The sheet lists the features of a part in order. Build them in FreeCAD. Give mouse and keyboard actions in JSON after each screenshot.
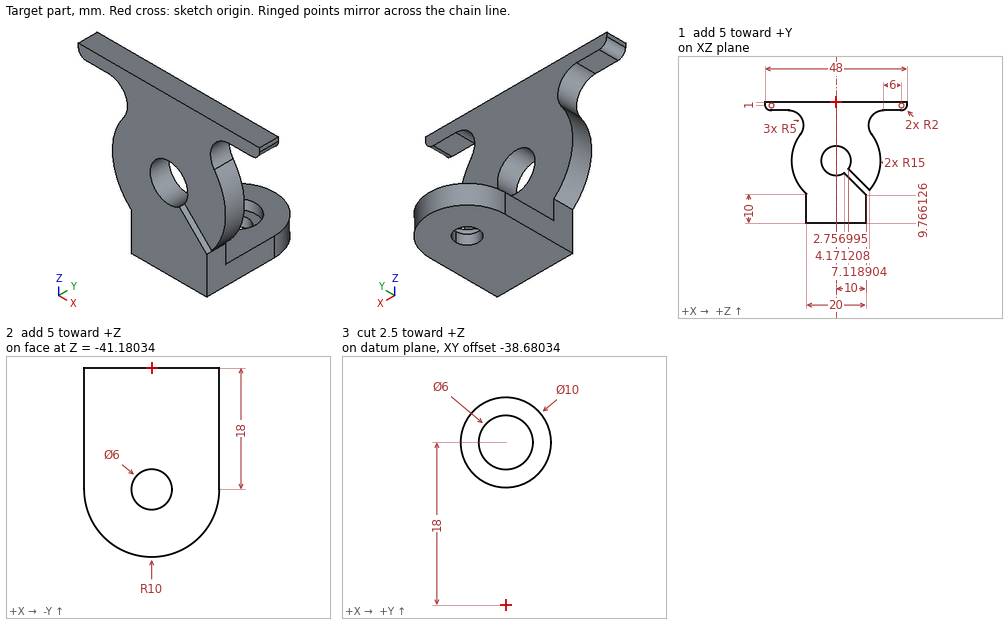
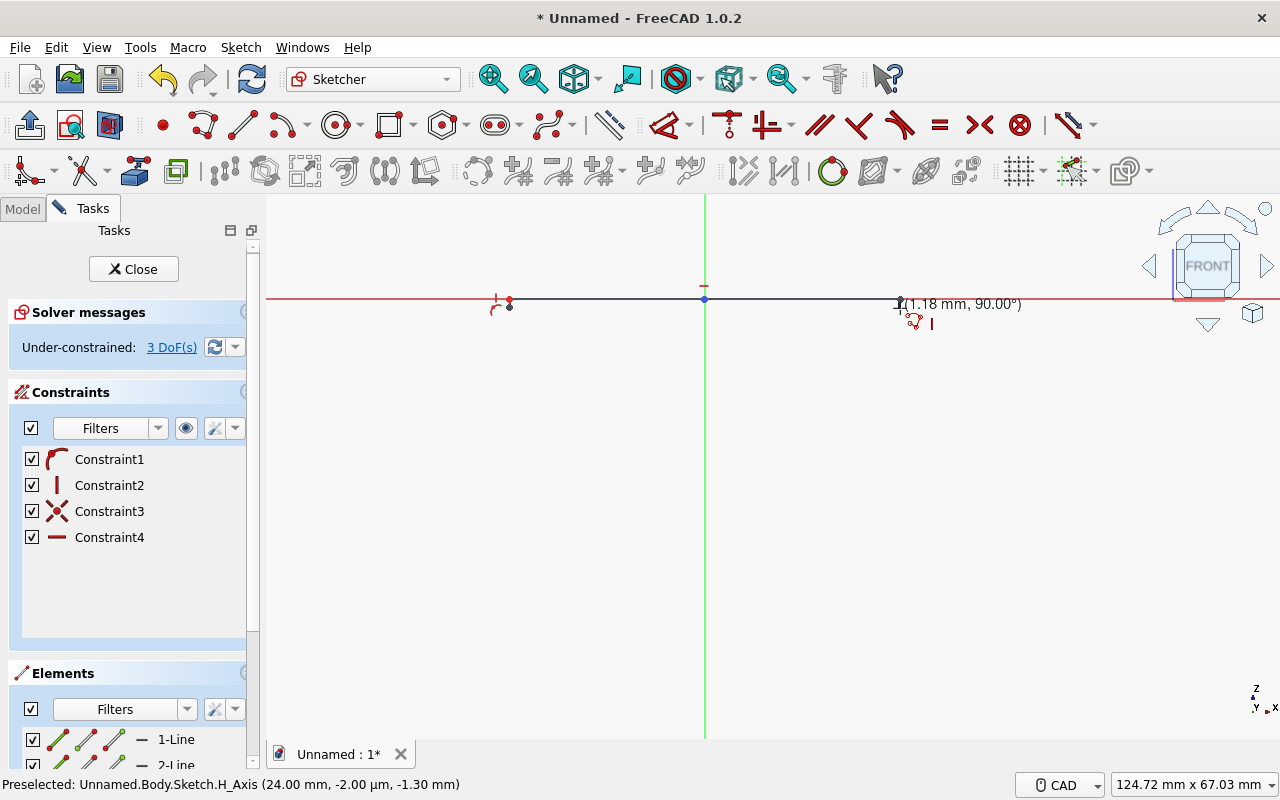
{"action": "scroll", "coordinate": [900, 308], "scroll_direction": "up", "scroll_amount": 4}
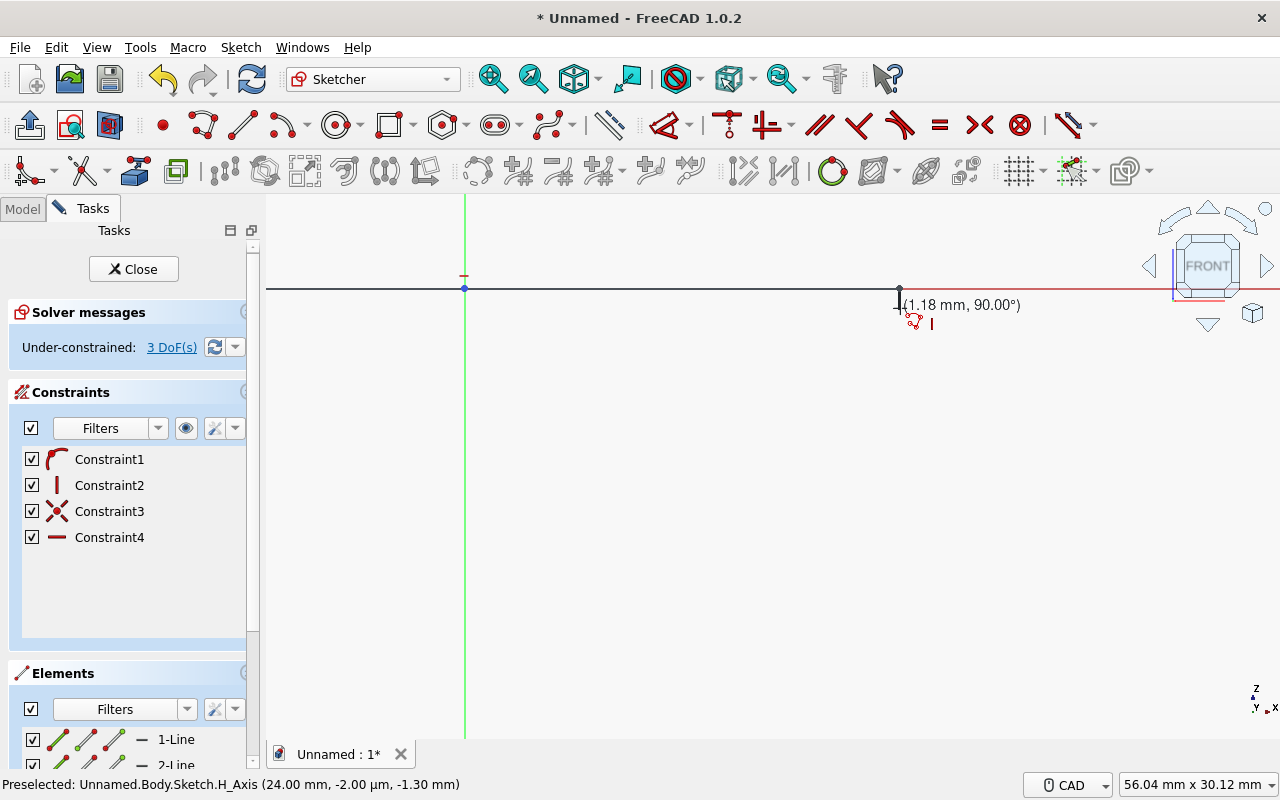
{"action": "left_click", "coordinate": [899, 307]}
{"action": "right_click", "coordinate": [899, 307]}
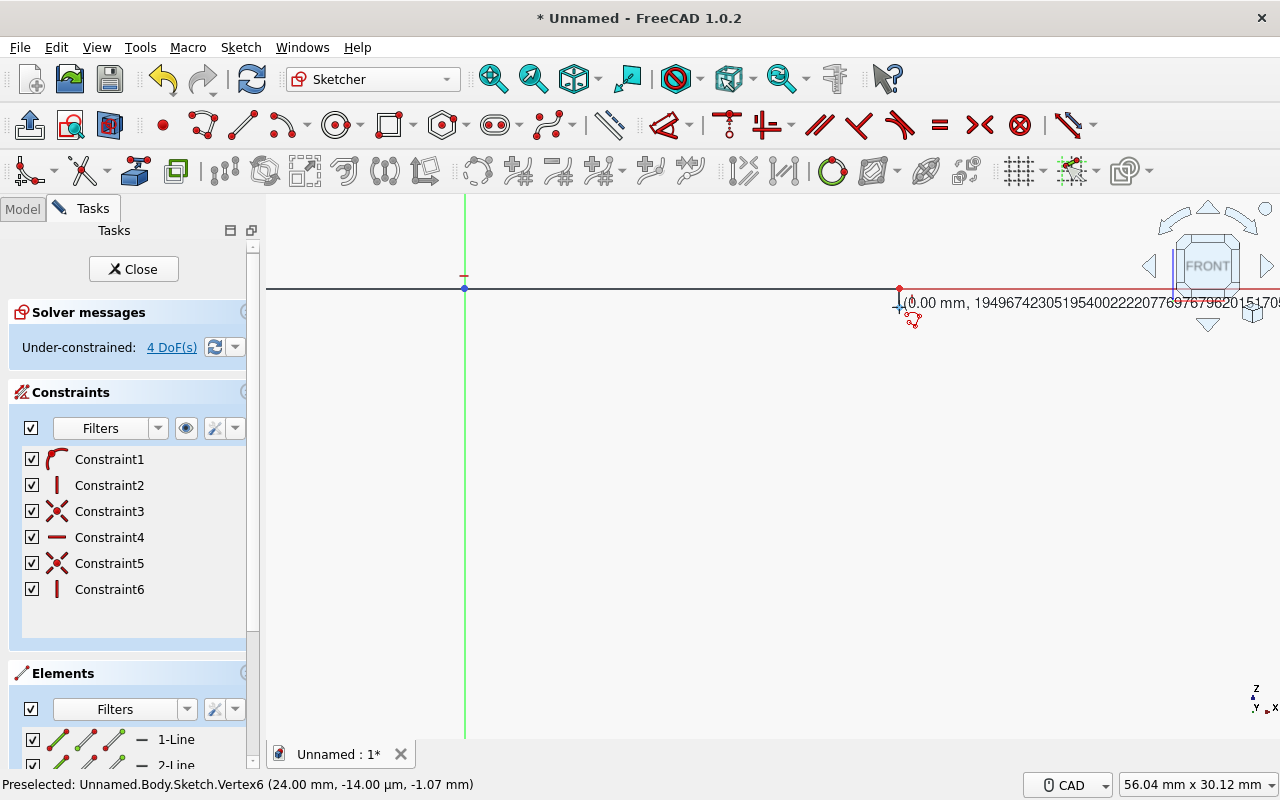
{"action": "key", "text": "g l"}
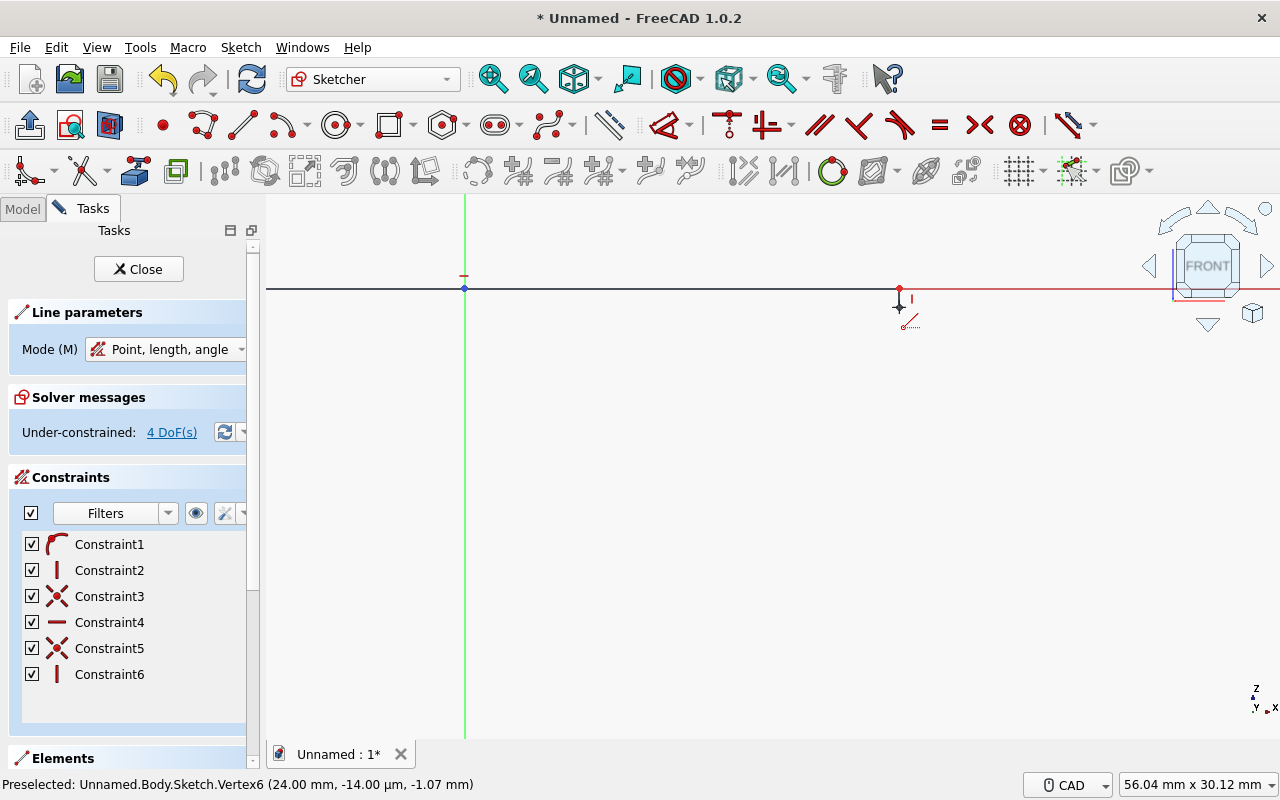
{"action": "left_click", "coordinate": [863, 343]}
{"action": "left_click", "coordinate": [754, 343]}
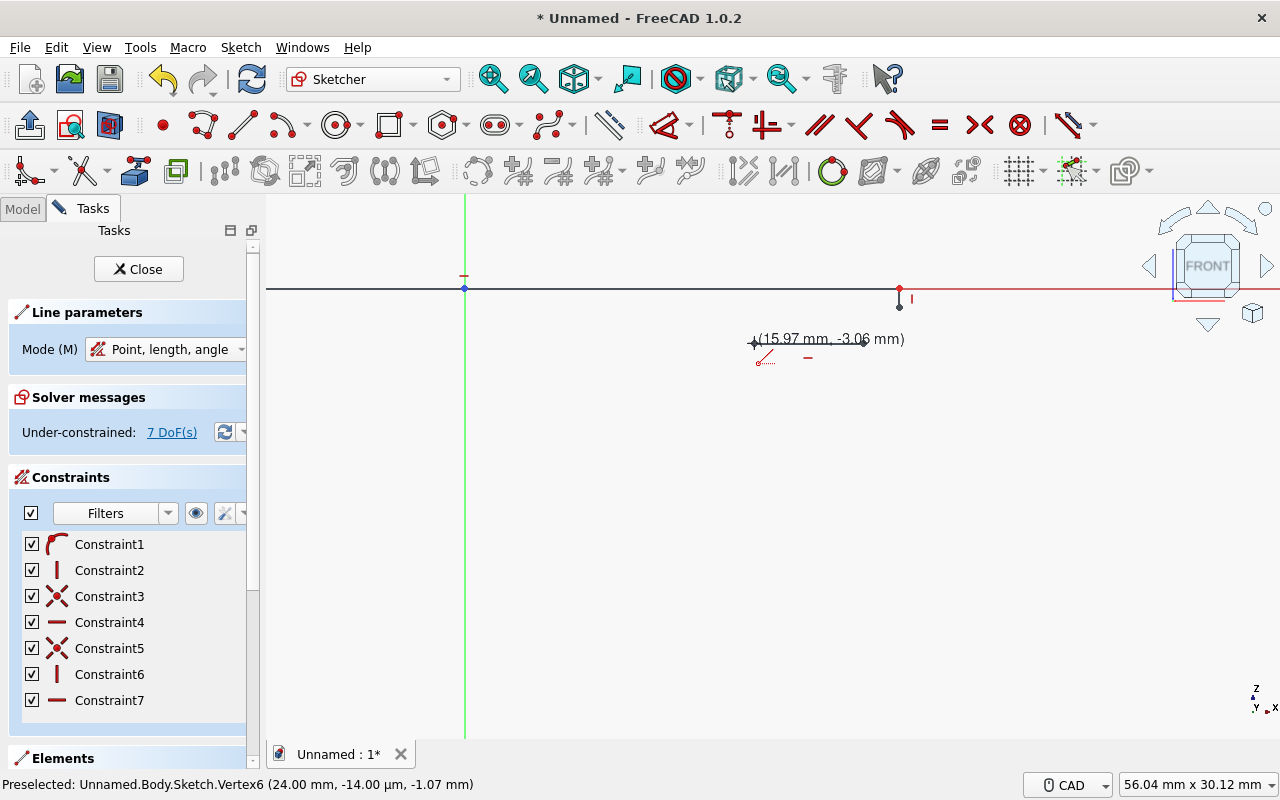
{"action": "scroll", "coordinate": [900, 308], "scroll_direction": "down", "scroll_amount": 4}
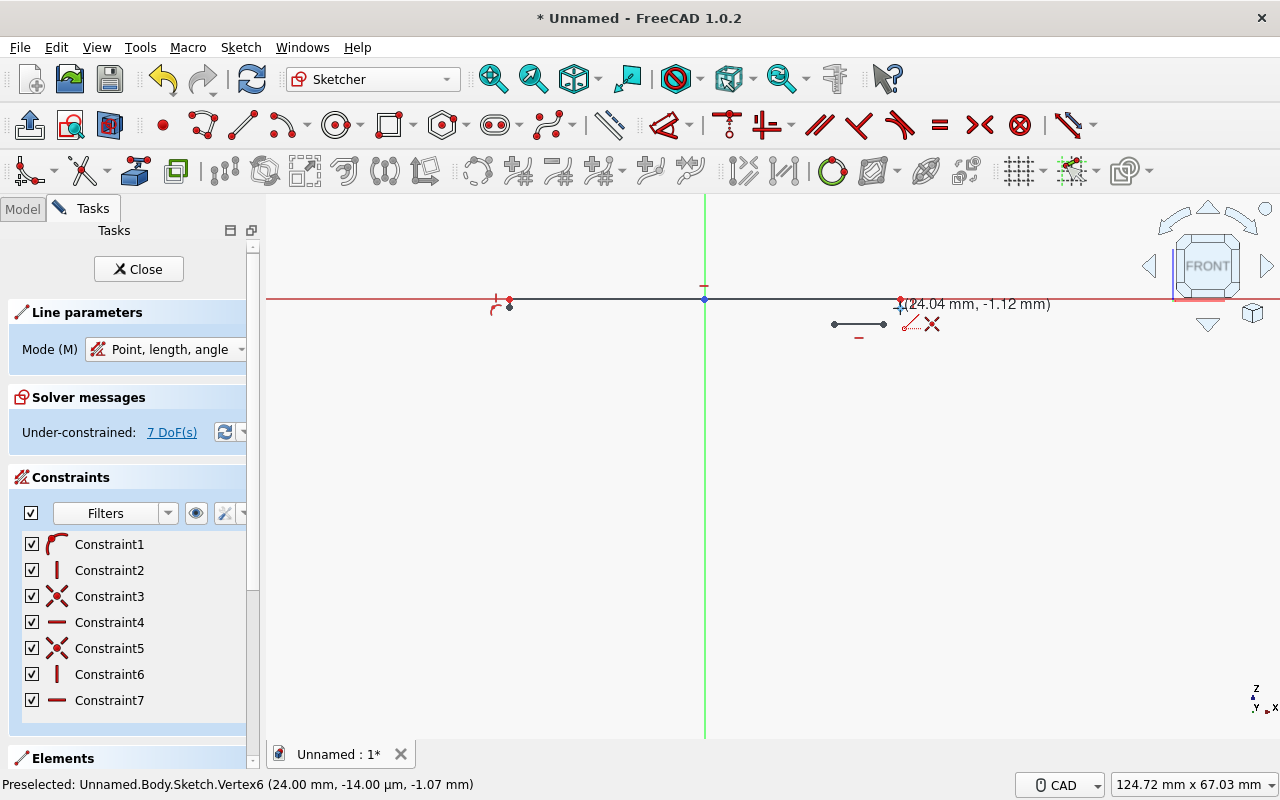
{"action": "left_click", "coordinate": [797, 542]}
{"action": "left_click", "coordinate": [739, 484]}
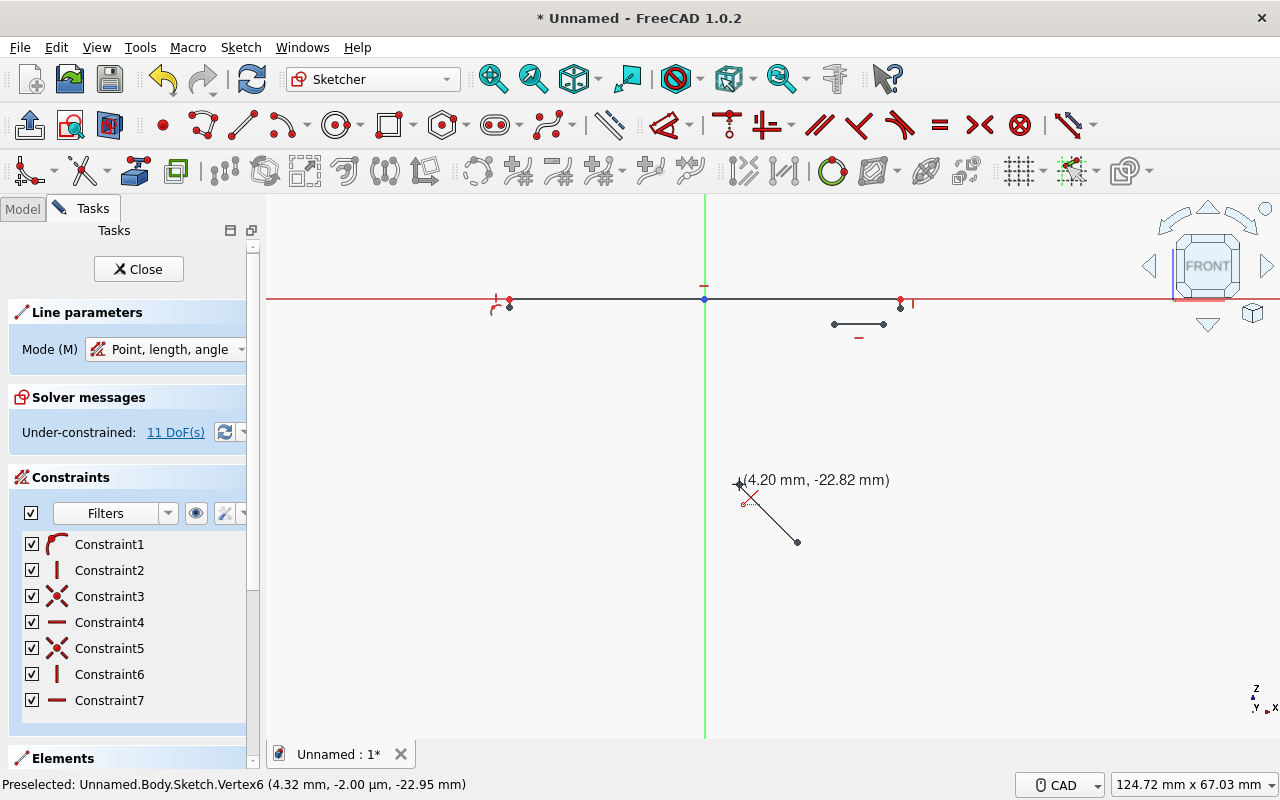
{"action": "key", "text": "g m"}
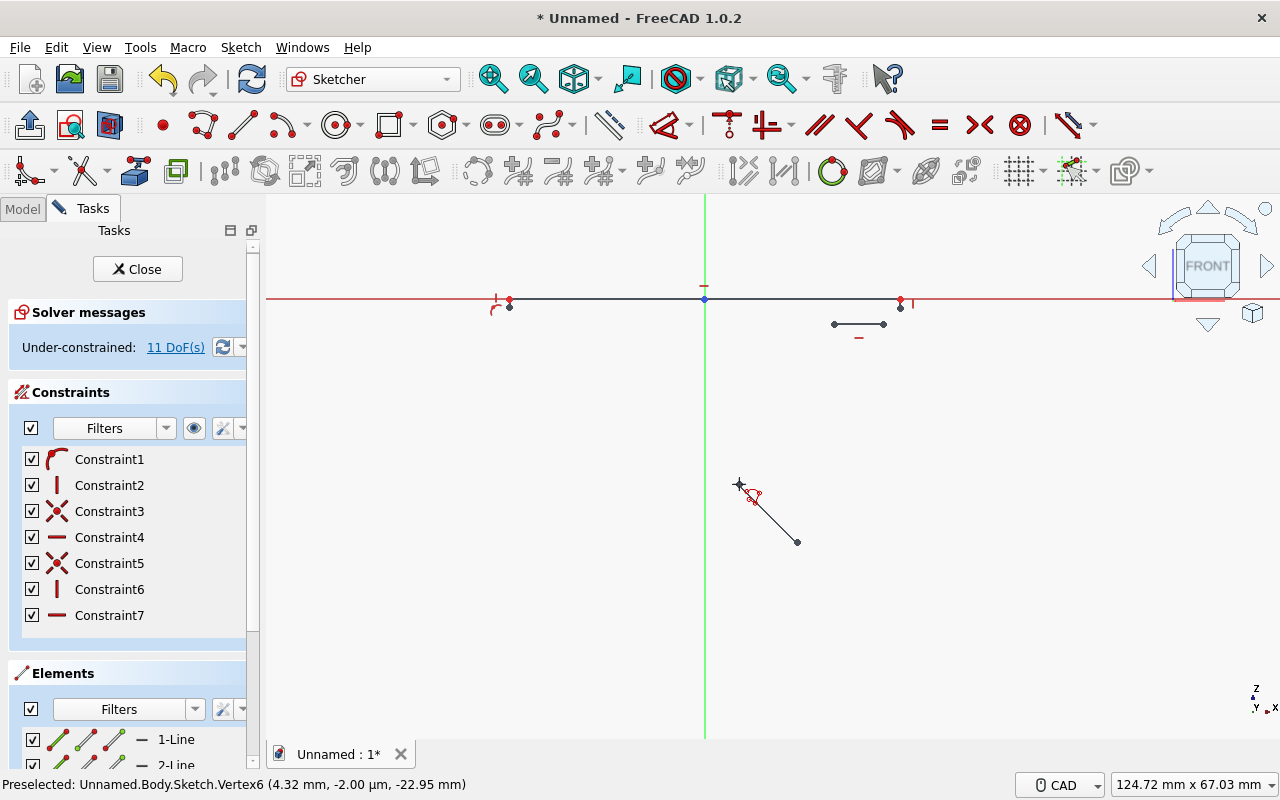
{"action": "left_click", "coordinate": [727, 496]}
{"action": "left_click", "coordinate": [786, 555]}
{"action": "left_click", "coordinate": [786, 634]}
{"action": "left_click", "coordinate": [624, 634]}
{"action": "left_click", "coordinate": [624, 553]}
{"action": "right_click", "coordinate": [624, 553]}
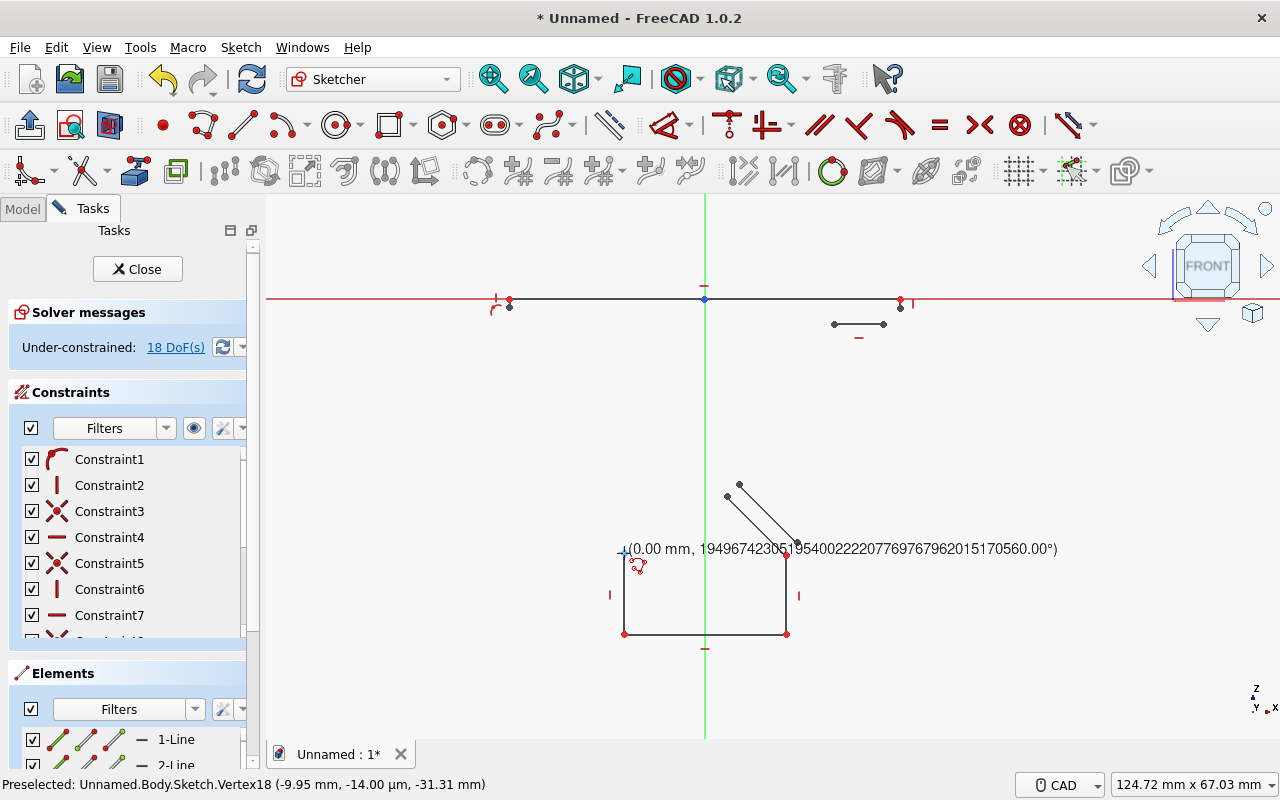
{"action": "left_click", "coordinate": [244, 126]}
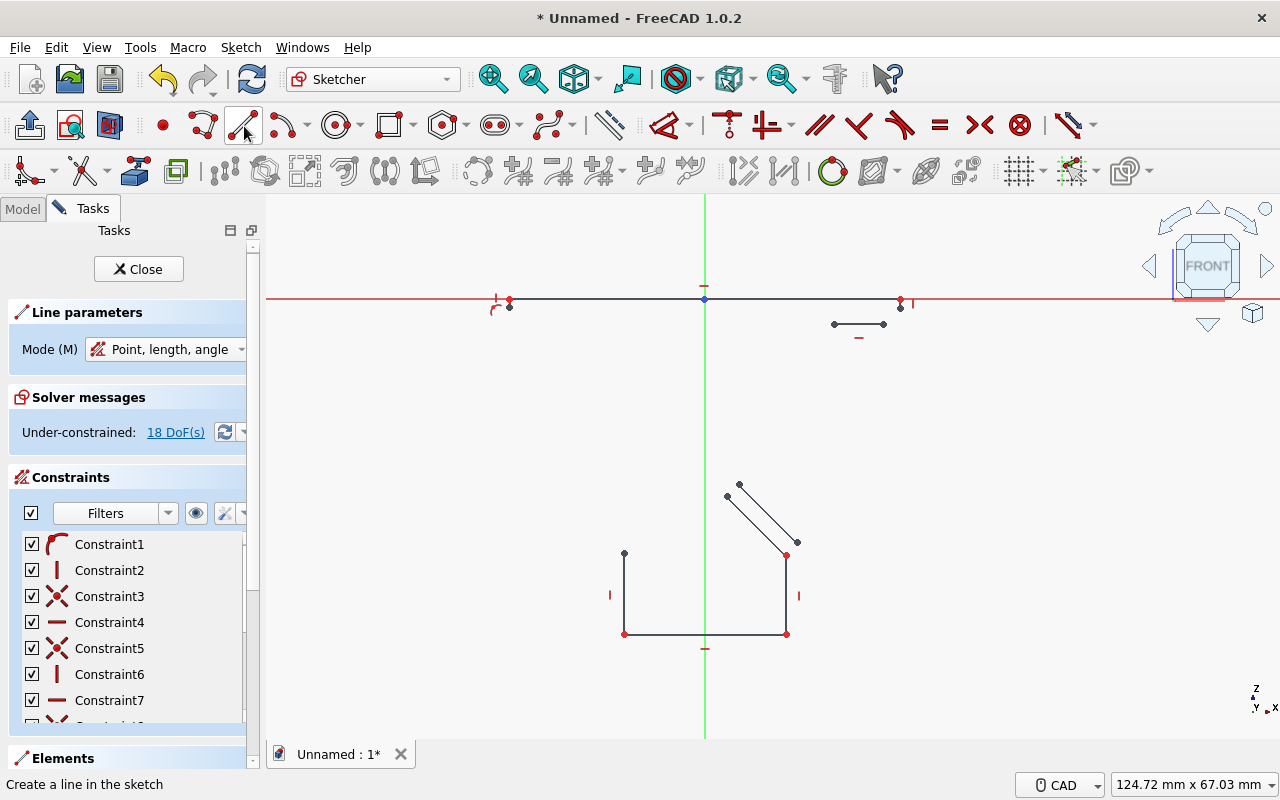
{"action": "left_click", "coordinate": [575, 324]}
{"action": "left_click", "coordinate": [526, 324]}